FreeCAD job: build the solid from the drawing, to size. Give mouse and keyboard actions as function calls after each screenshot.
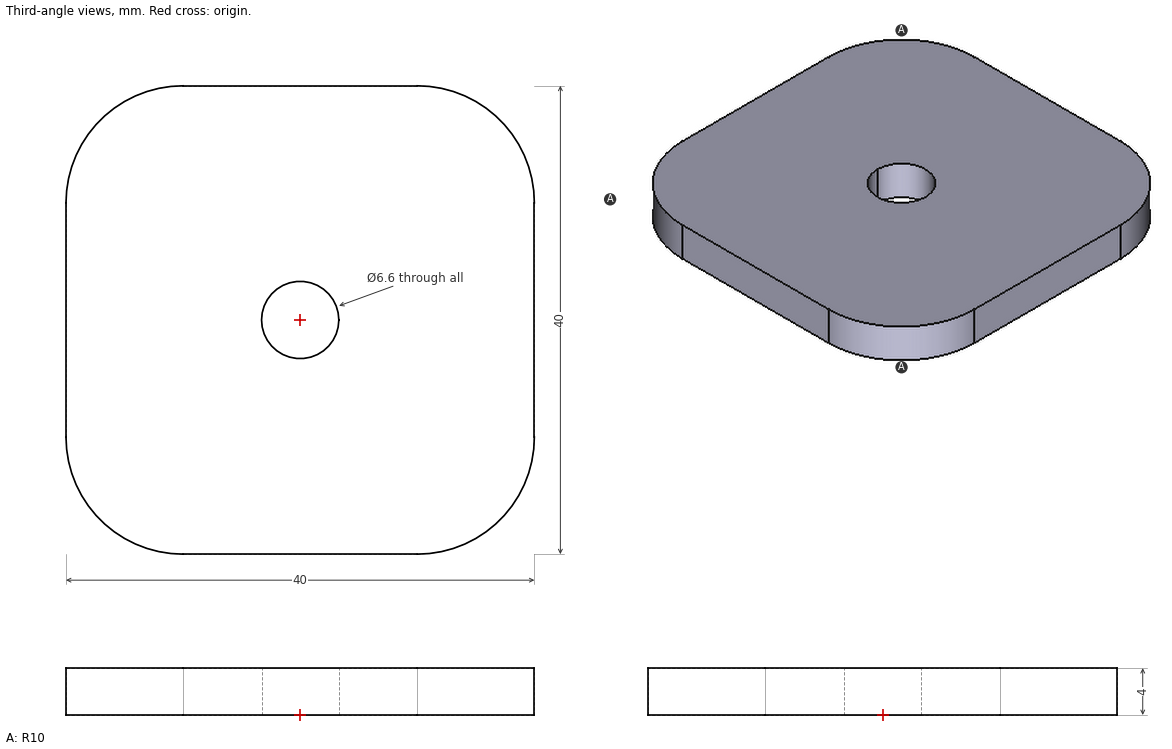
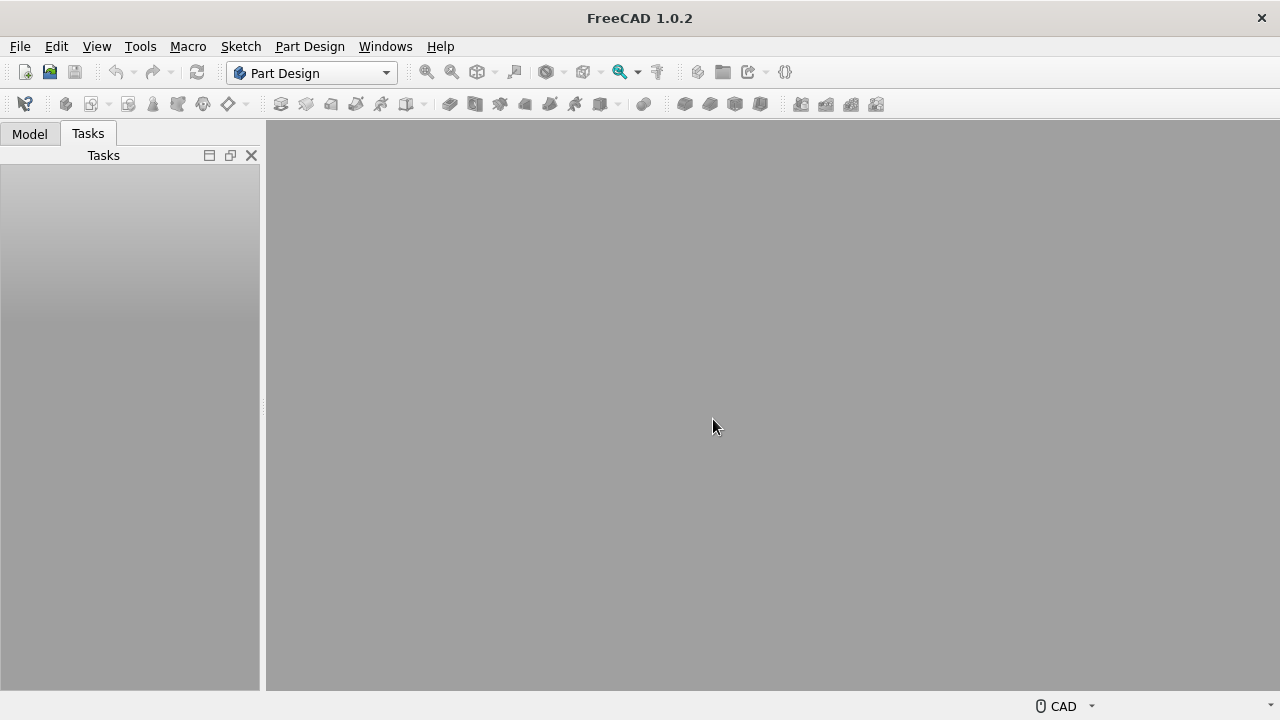
key(ctrl+n)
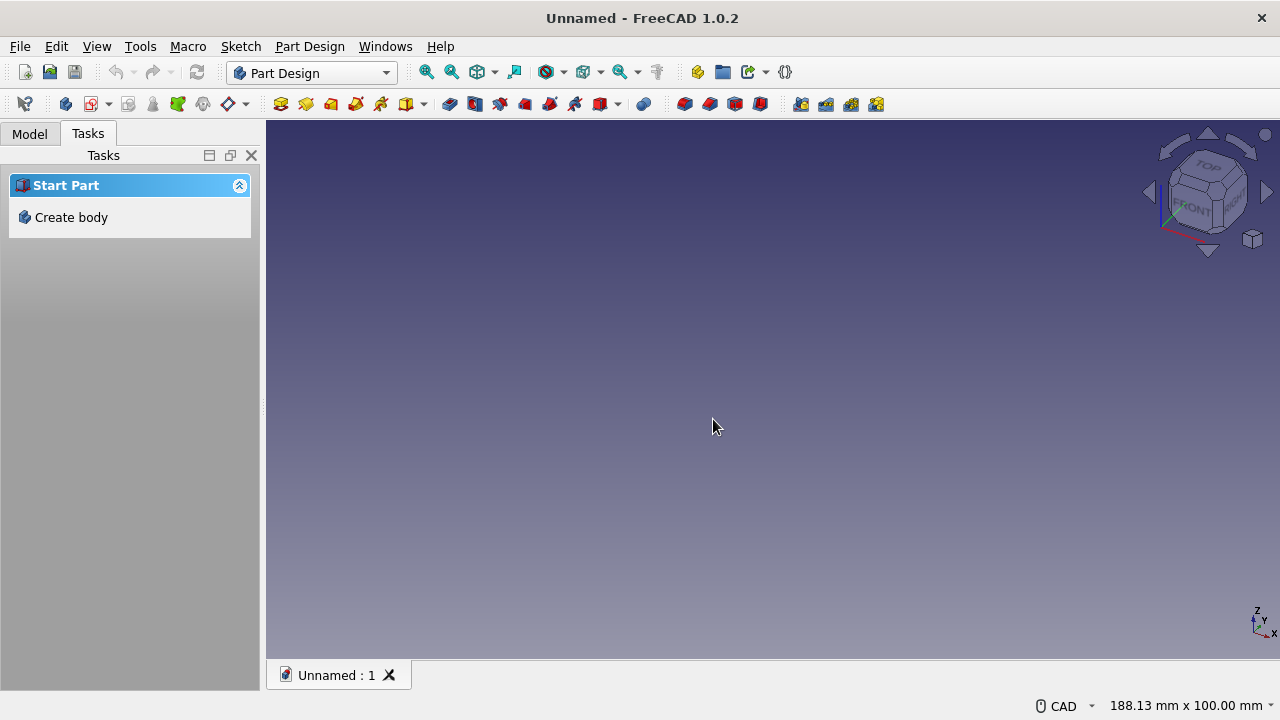
click(90, 104)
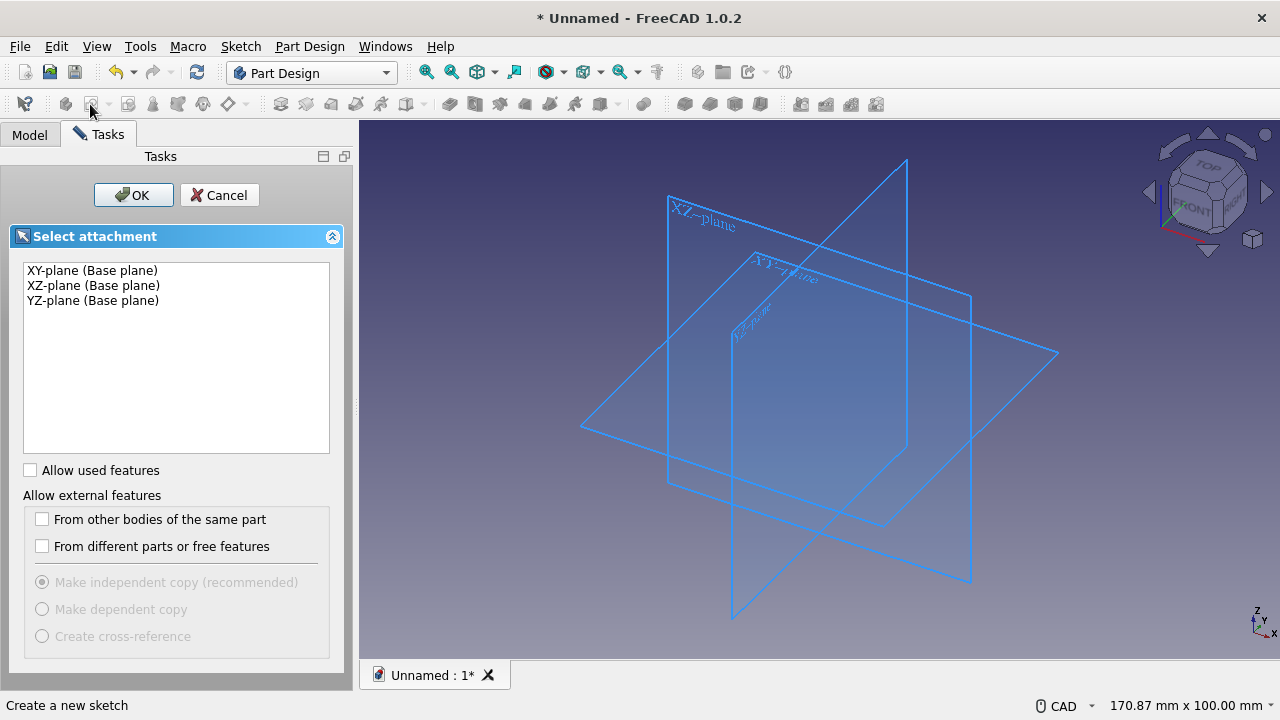
click(84, 270)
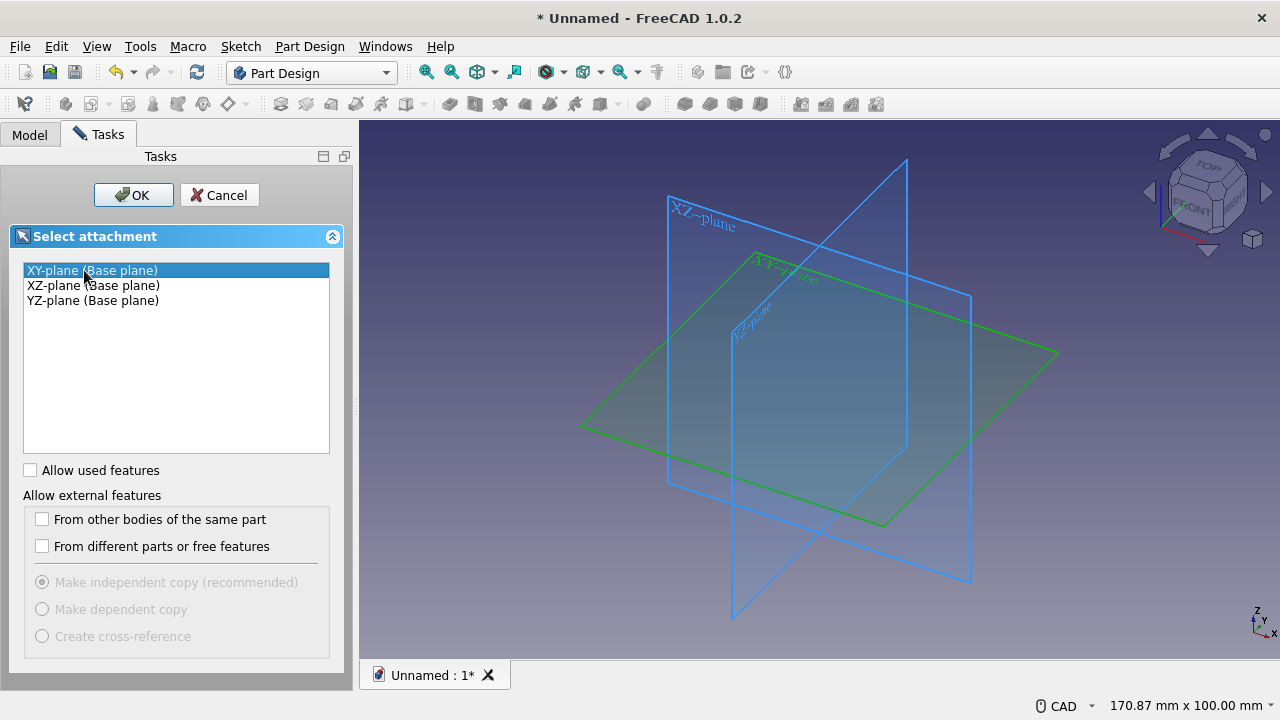
click(134, 195)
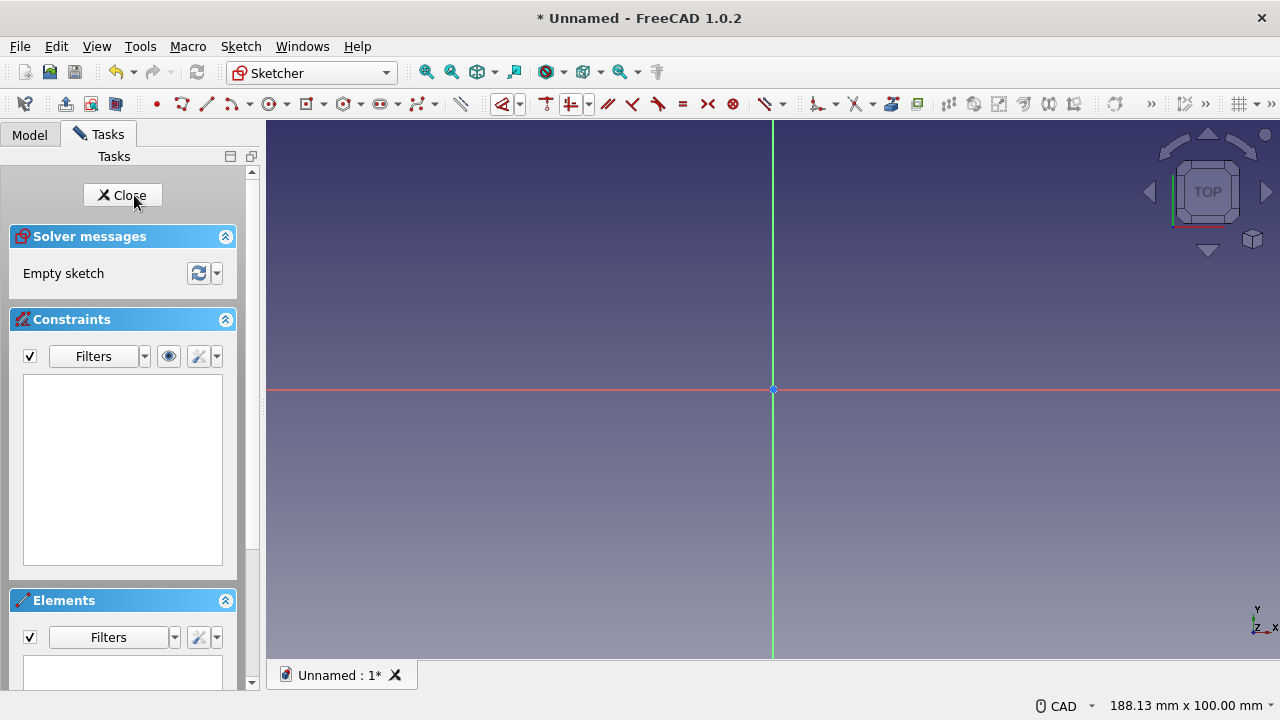
scroll(912, 390, up, 2)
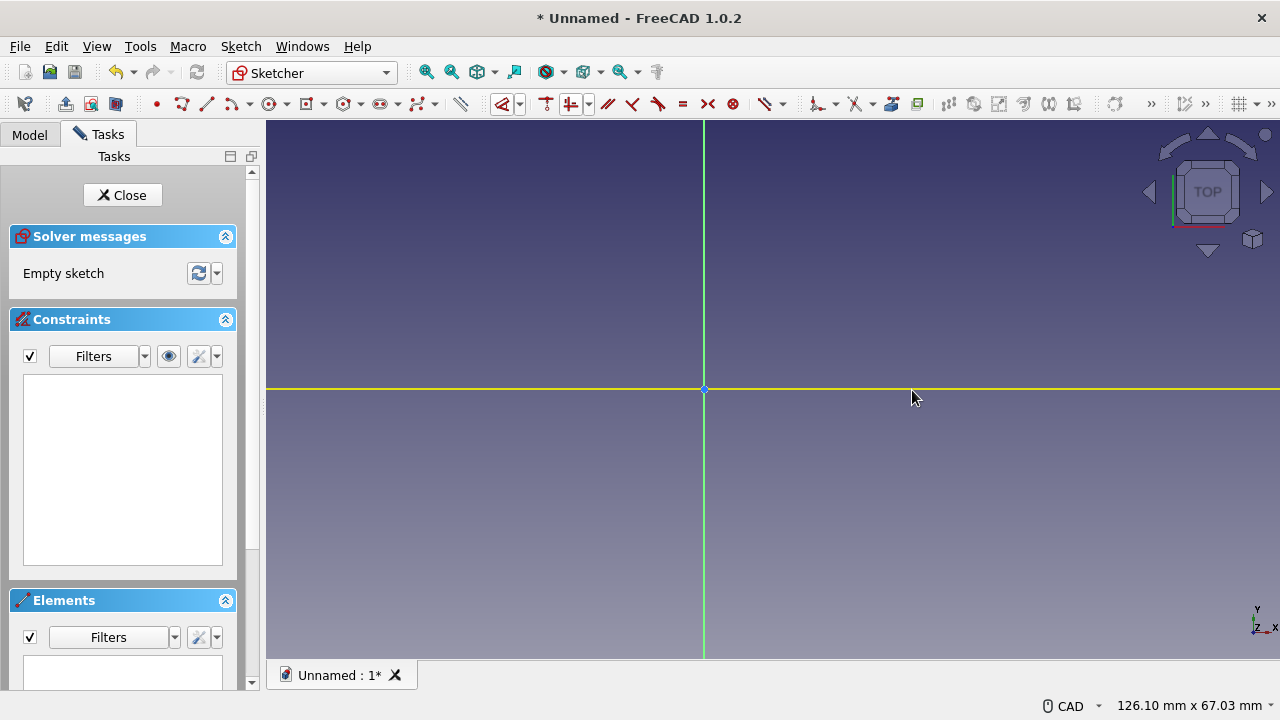
click(306, 104)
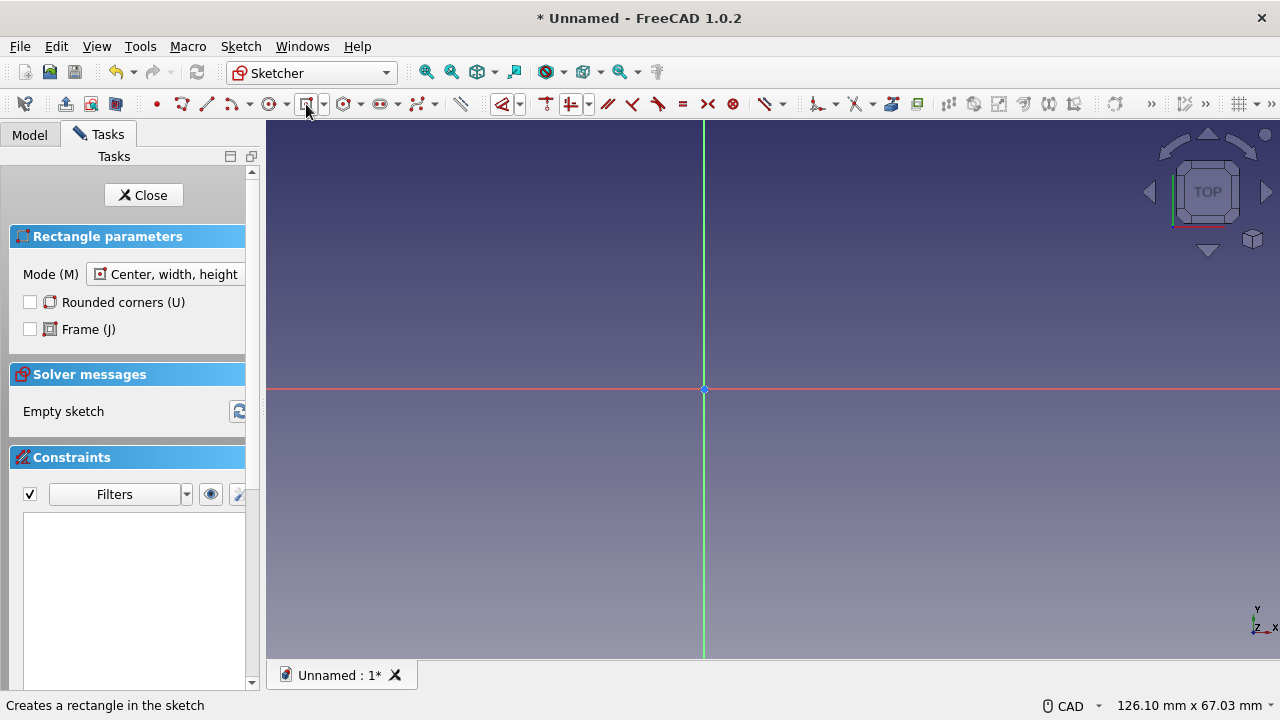
click(704, 389)
click(865, 228)
key(Escape)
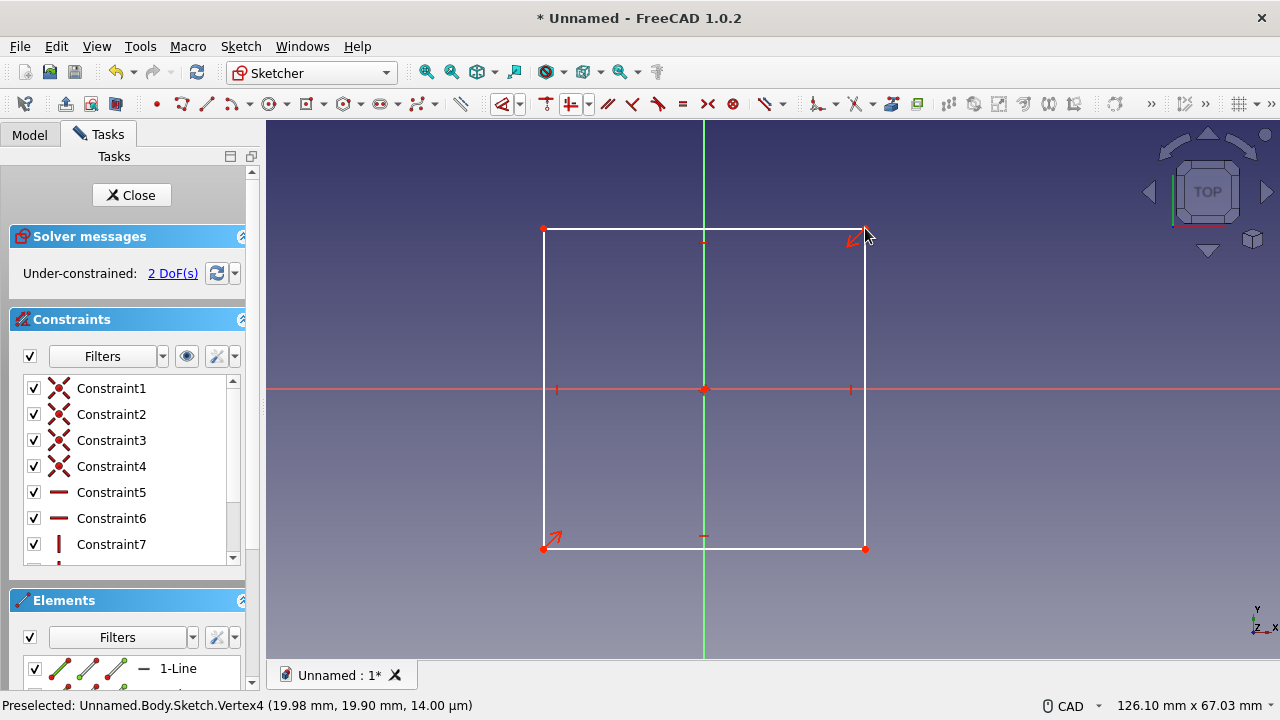
click(640, 549)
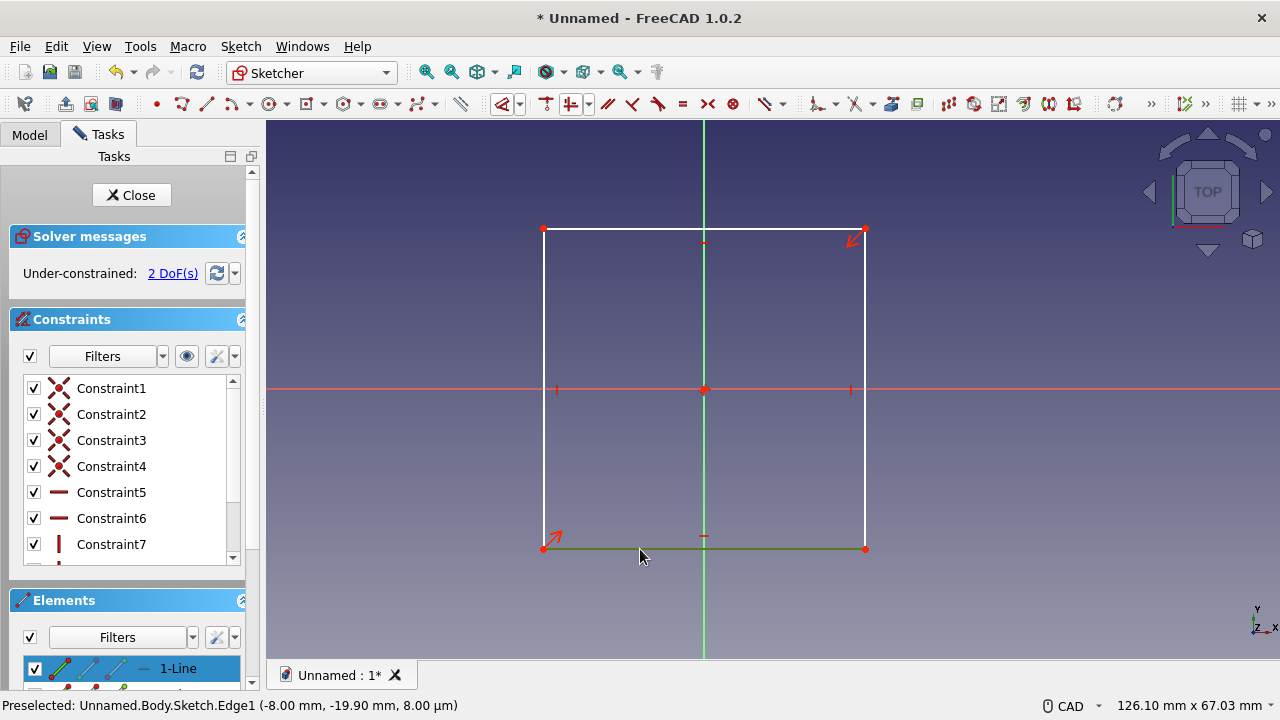
click(520, 104)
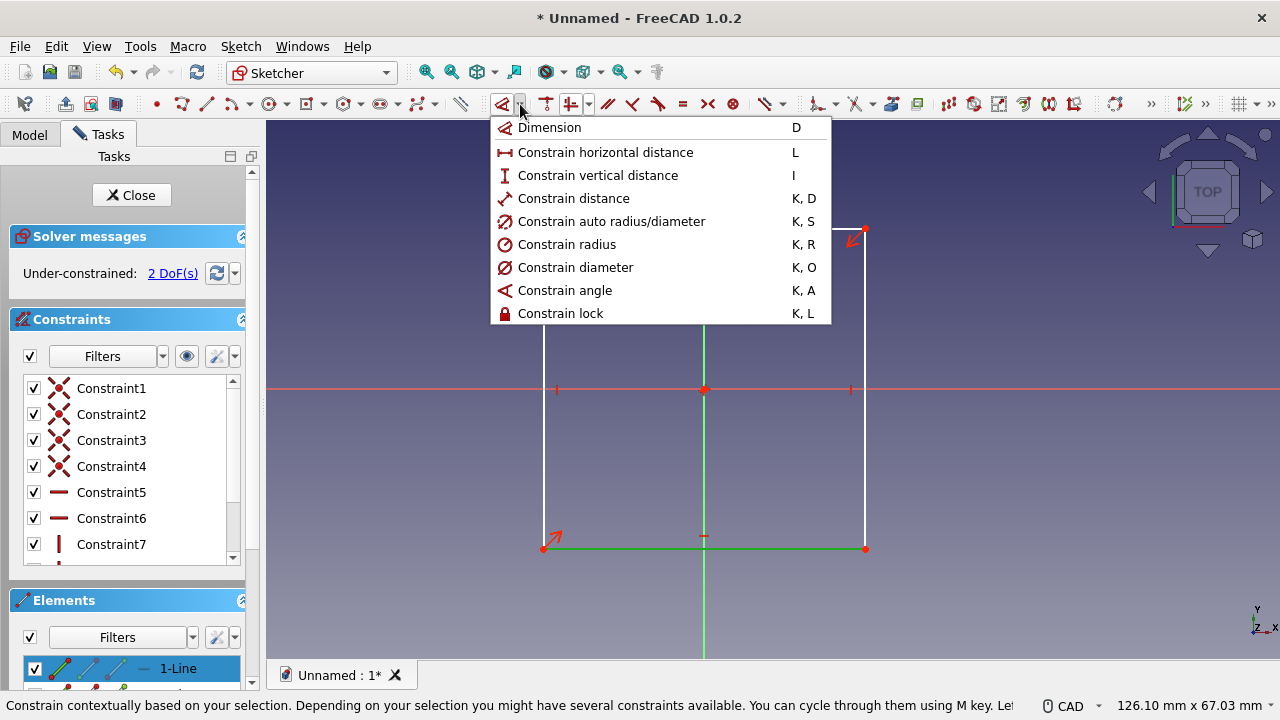
click(661, 152)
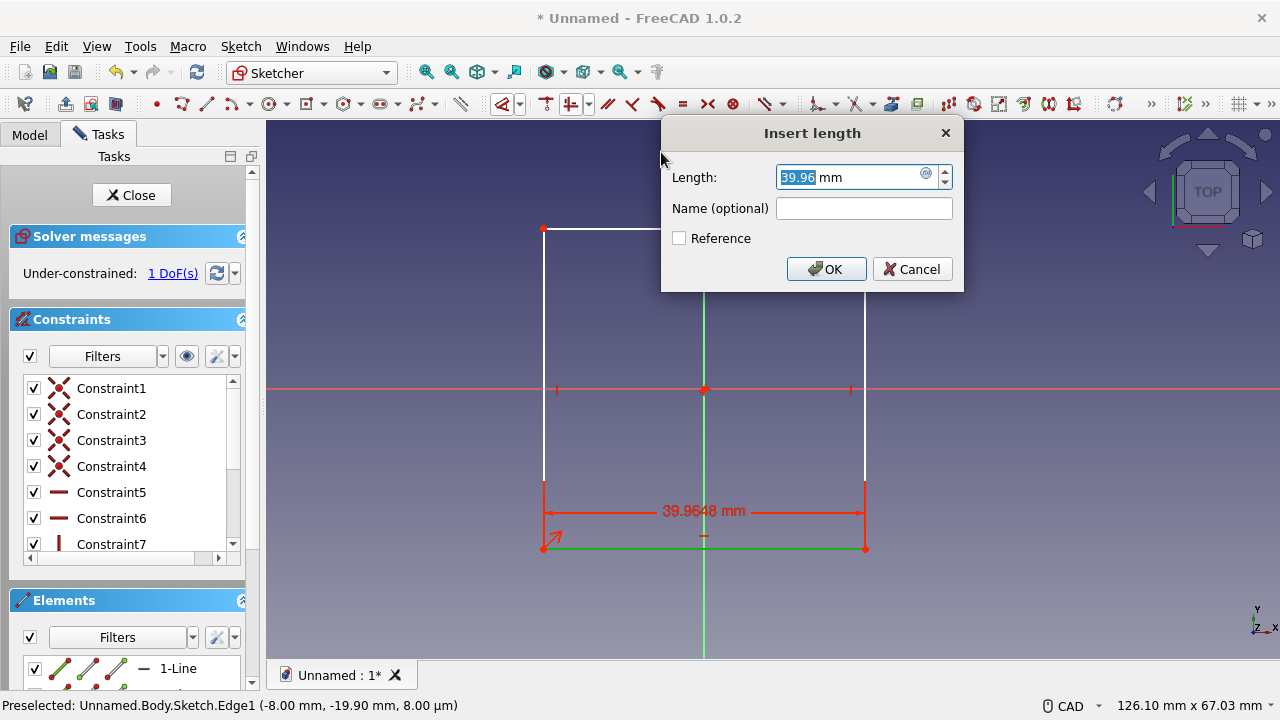
text(40)
key(Return)